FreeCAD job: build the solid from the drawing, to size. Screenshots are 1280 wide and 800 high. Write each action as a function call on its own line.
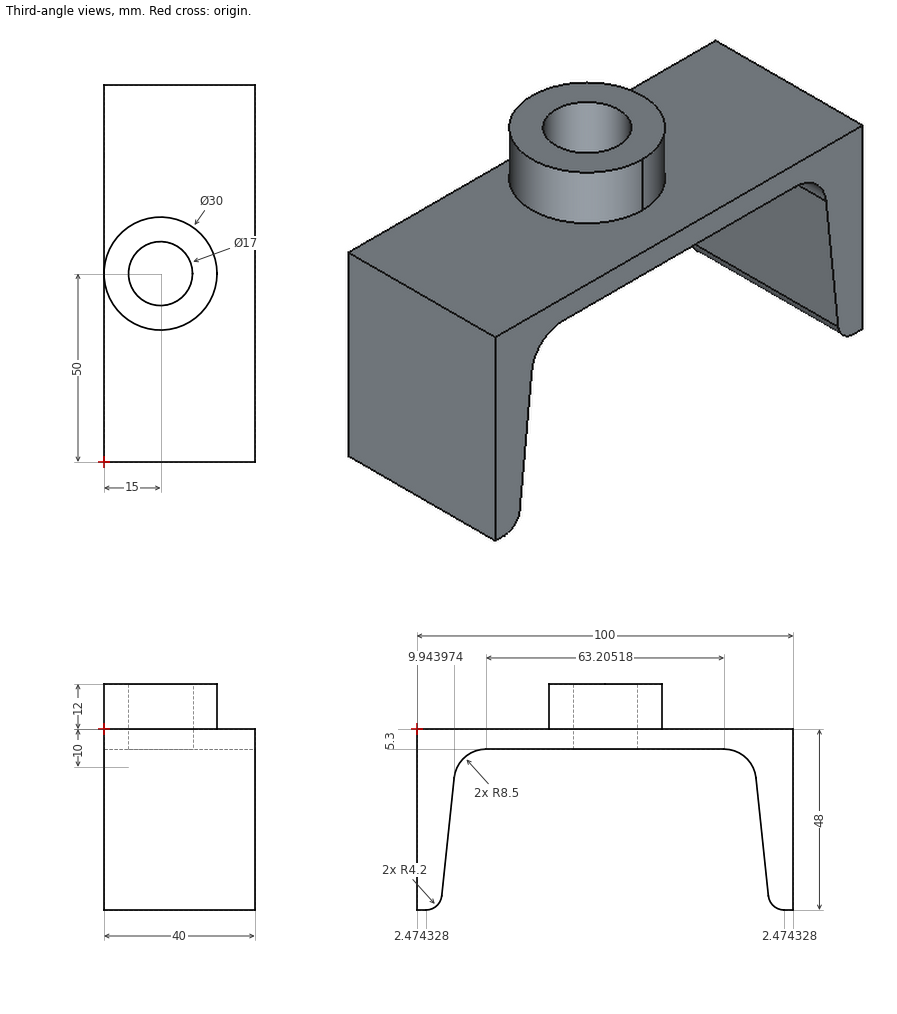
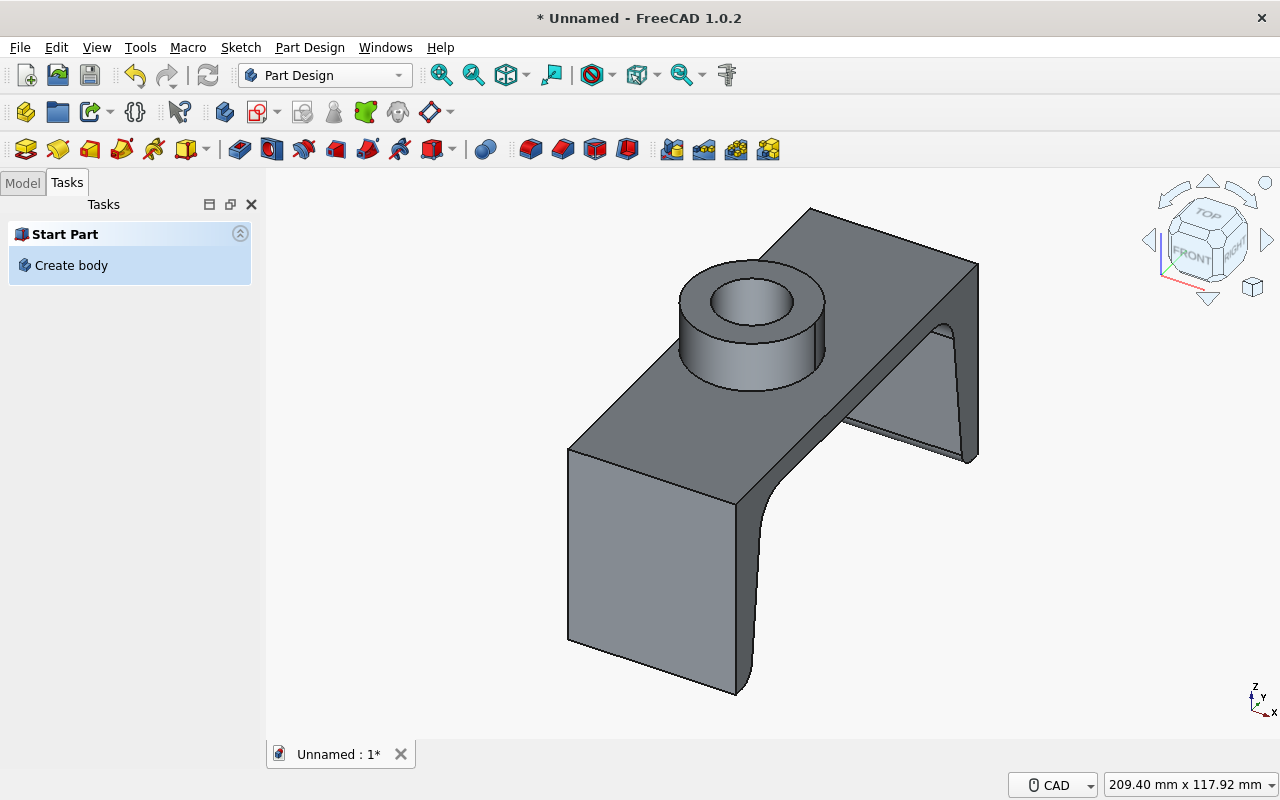
key(0)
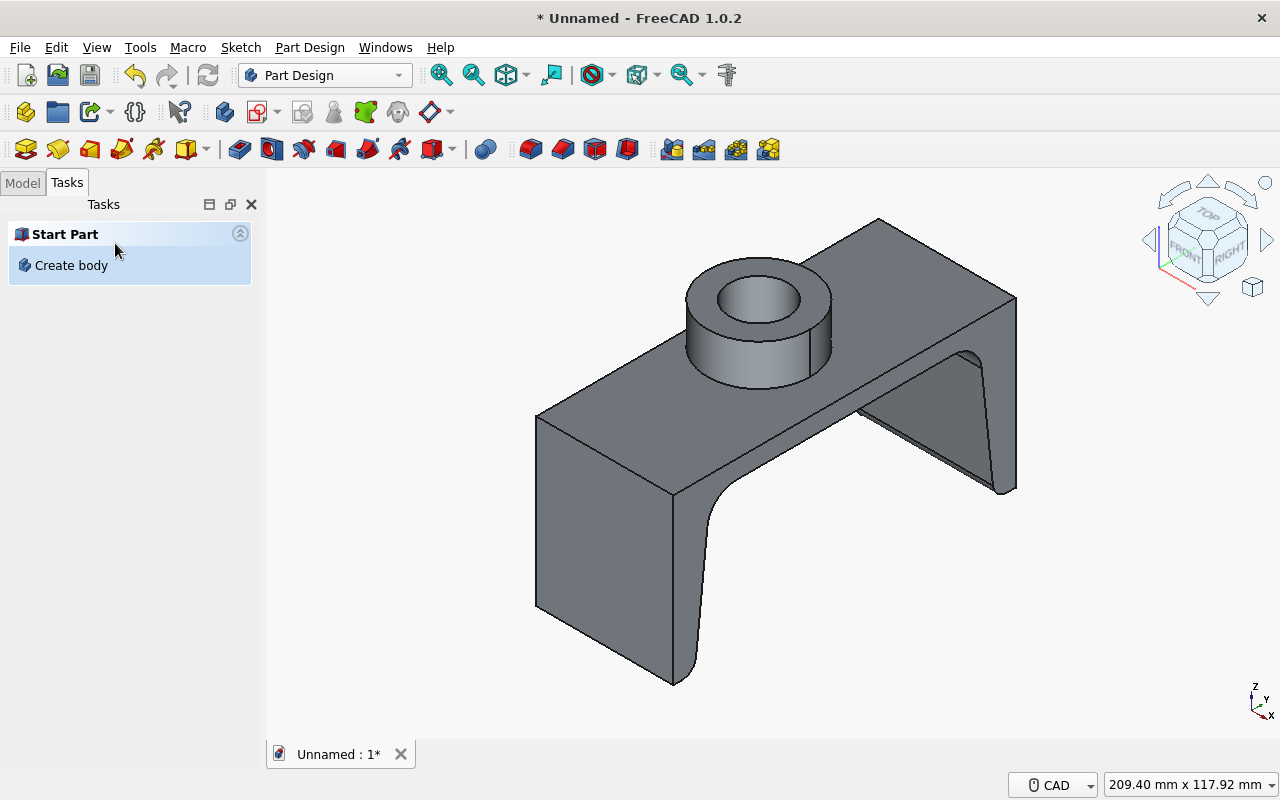
click(442, 76)